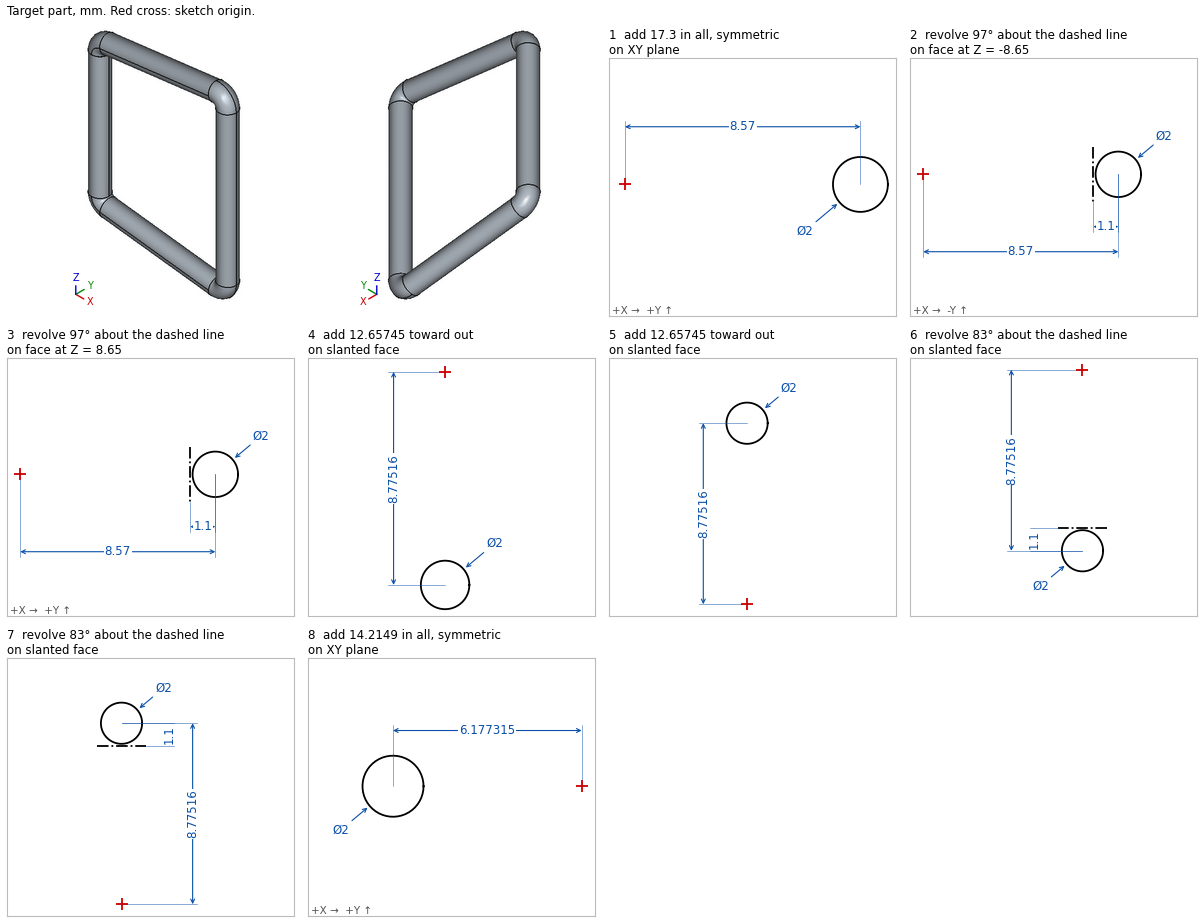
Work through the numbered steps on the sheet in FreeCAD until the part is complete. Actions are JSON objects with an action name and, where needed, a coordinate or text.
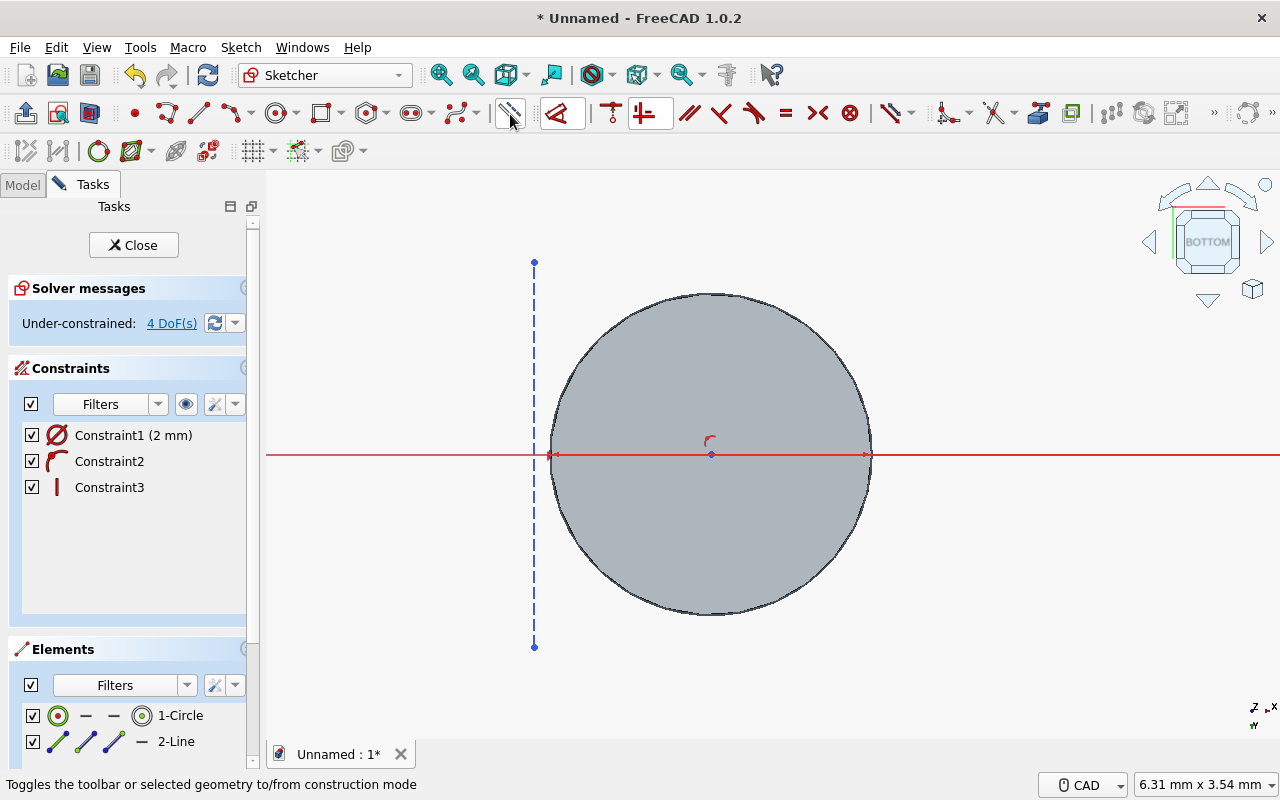
{"action": "left_click", "coordinate": [556, 114]}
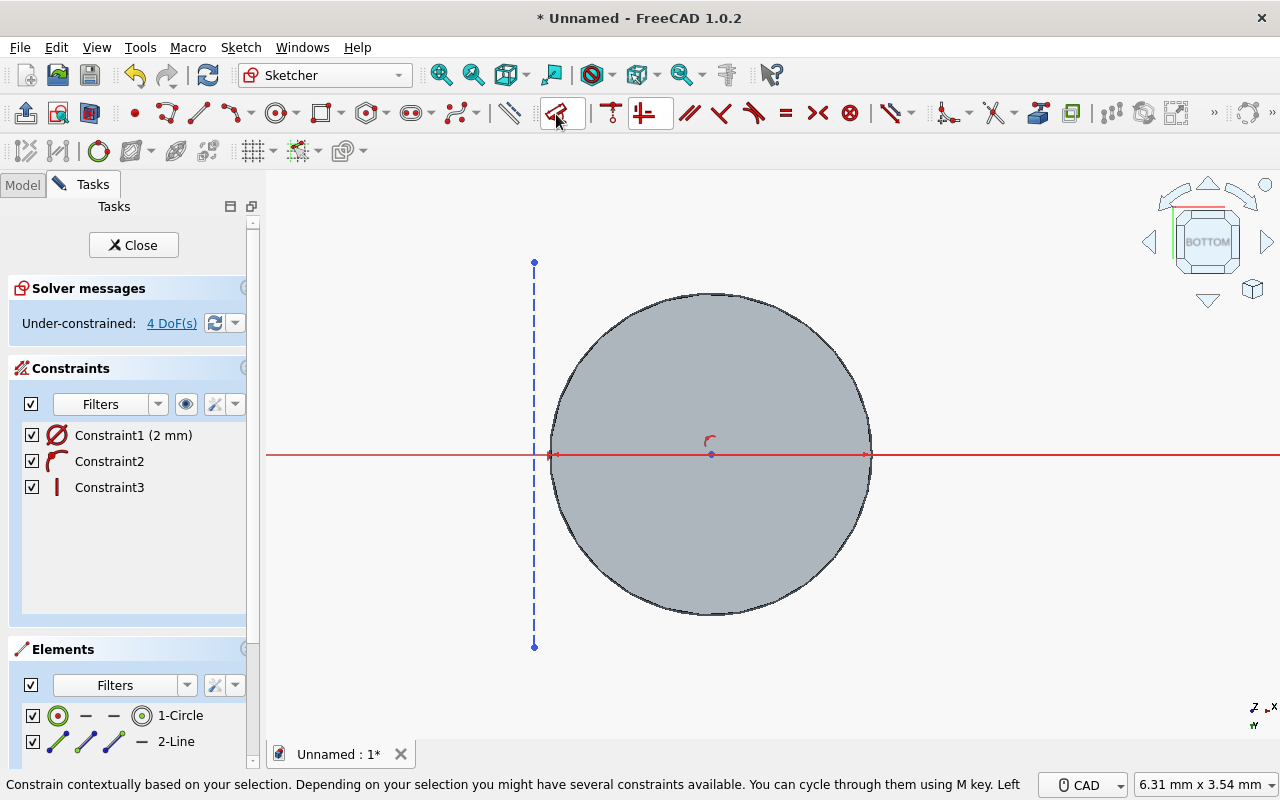
{"action": "scroll", "coordinate": [711, 454], "scroll_direction": "up", "scroll_amount": 4}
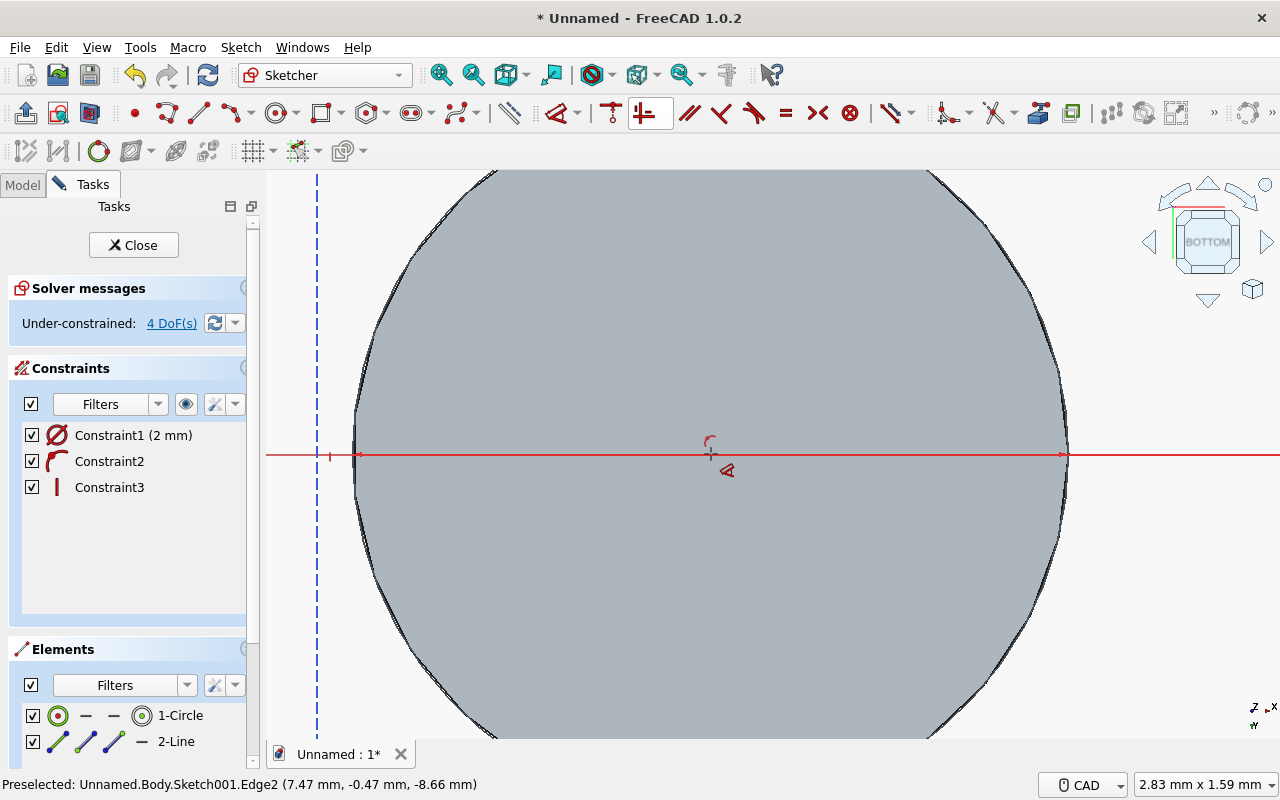
{"action": "left_click", "coordinate": [710, 454]}
{"action": "left_click", "coordinate": [502, 488]}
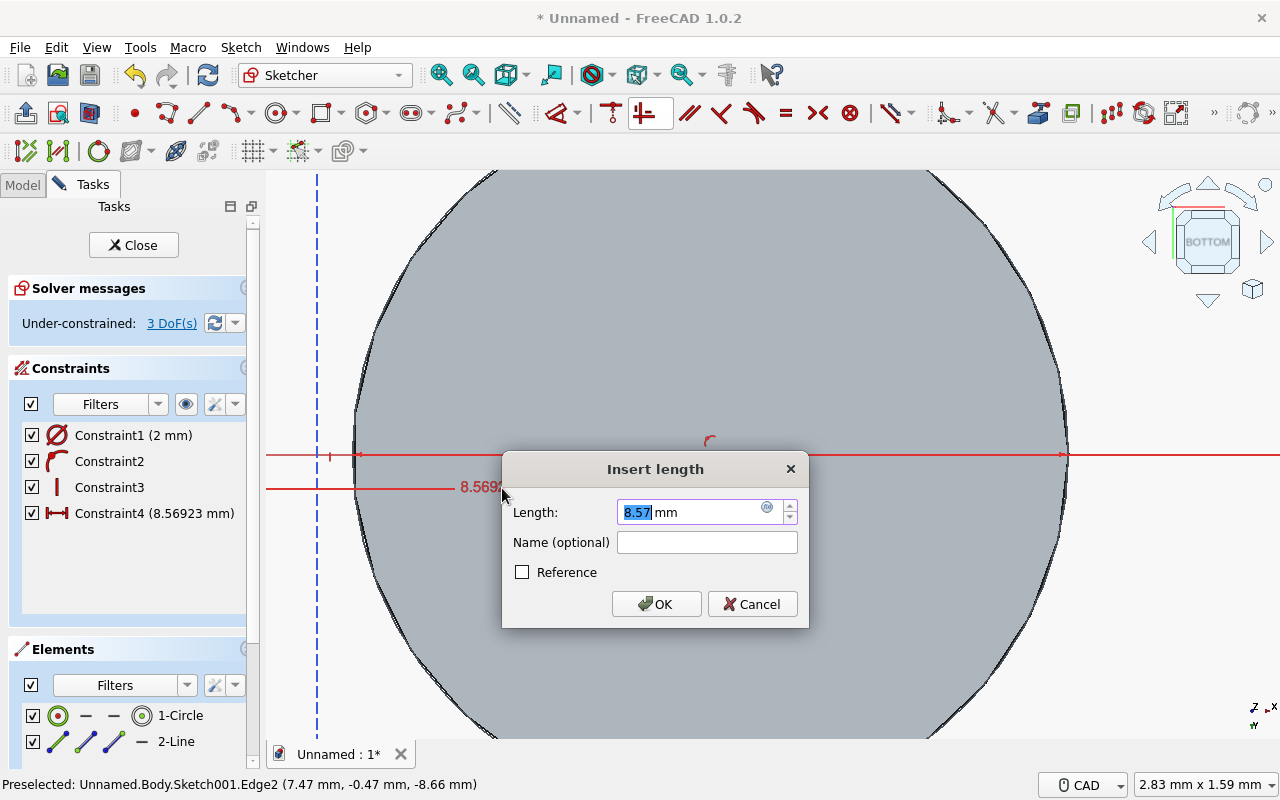
{"action": "type", "text": "8.57"}
{"action": "key", "text": "Return"}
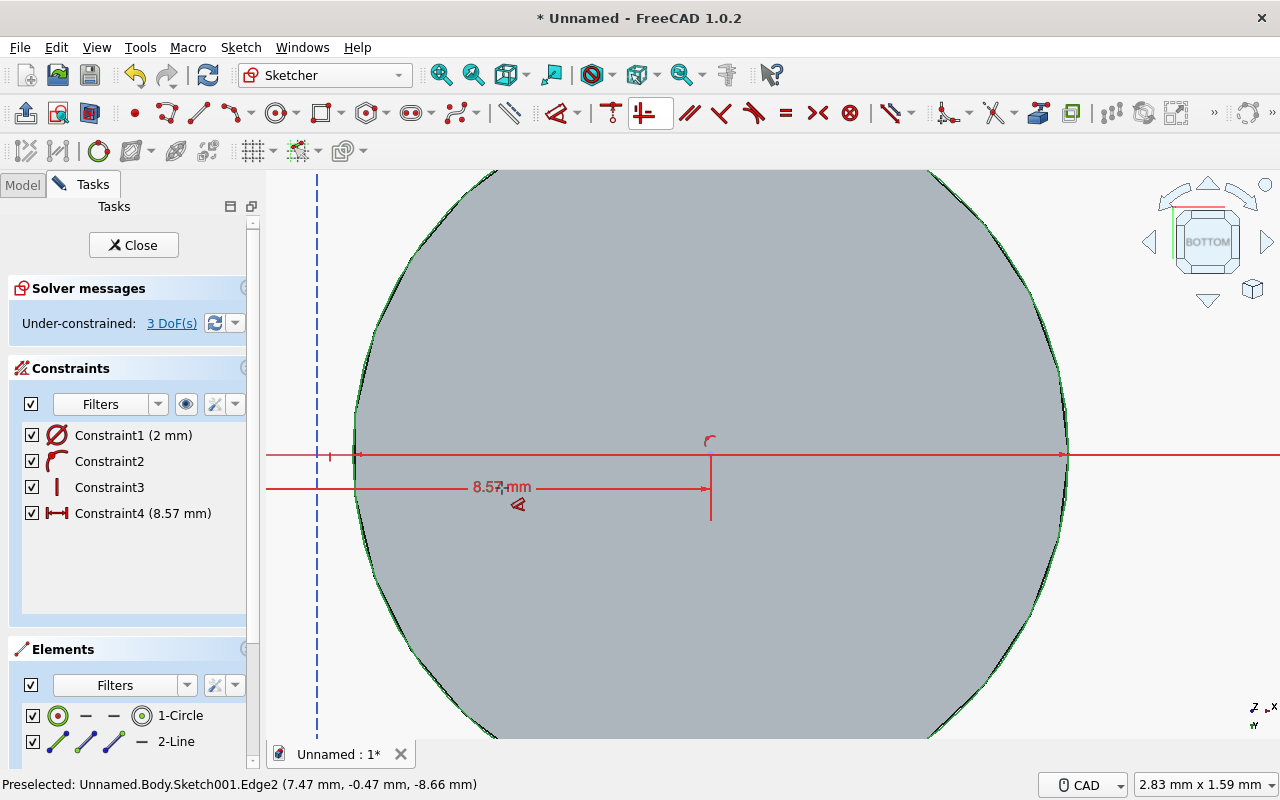
{"action": "scroll", "coordinate": [714, 454], "scroll_direction": "down", "scroll_amount": 4}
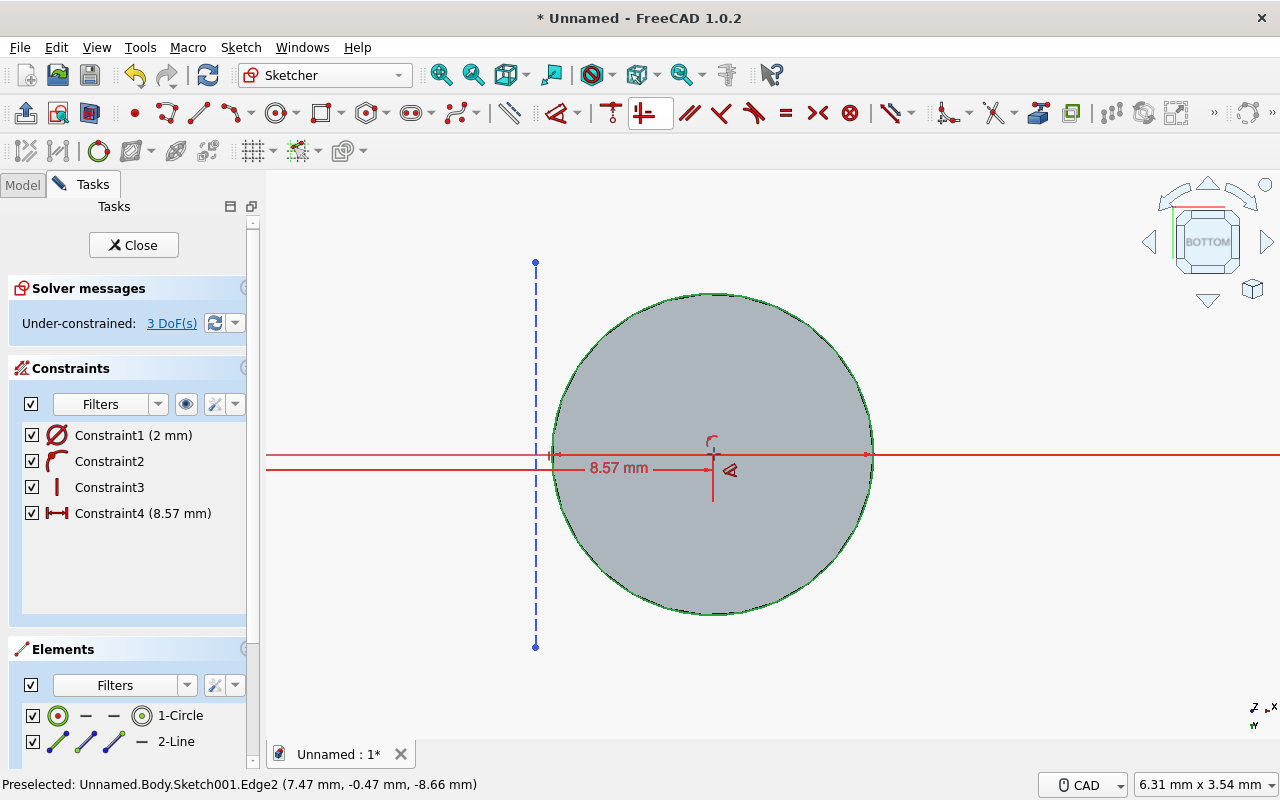
{"action": "left_click", "coordinate": [538, 650]}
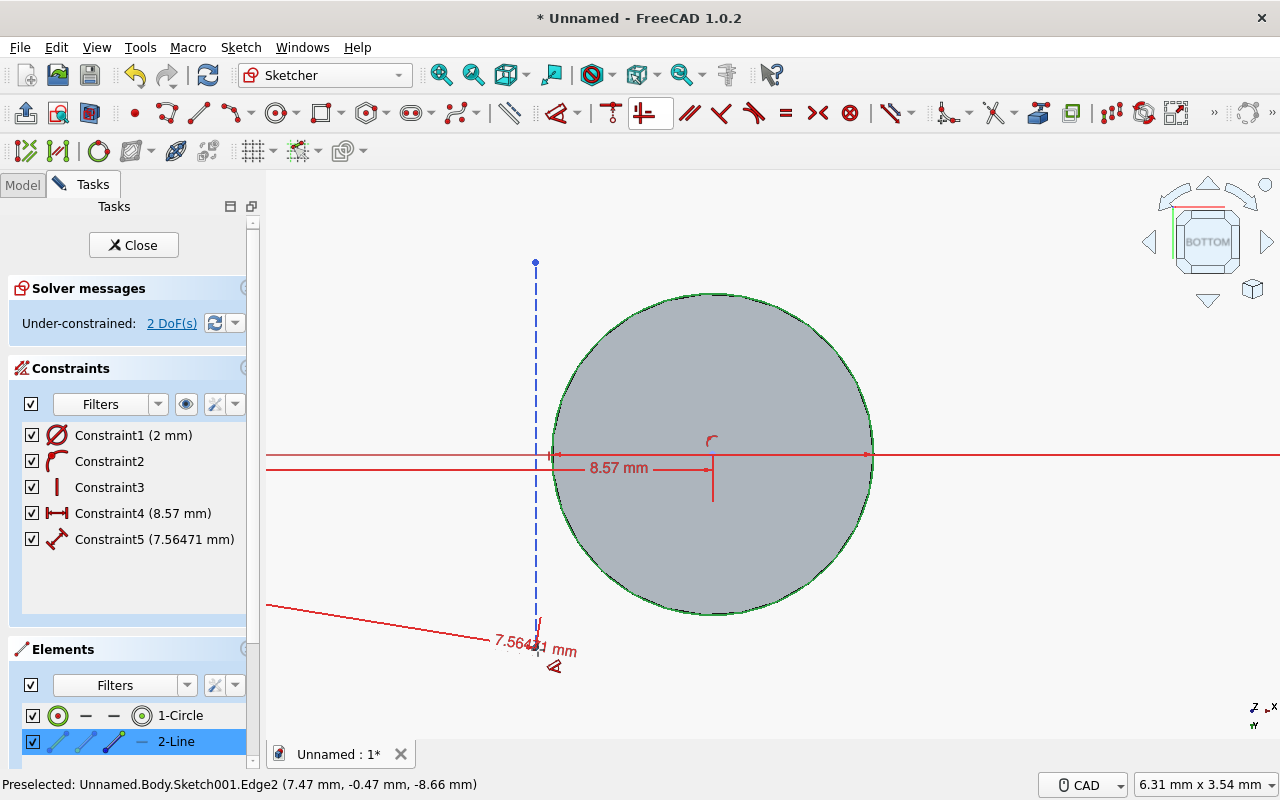
{"action": "left_click", "coordinate": [713, 454]}
{"action": "left_click", "coordinate": [624, 682]}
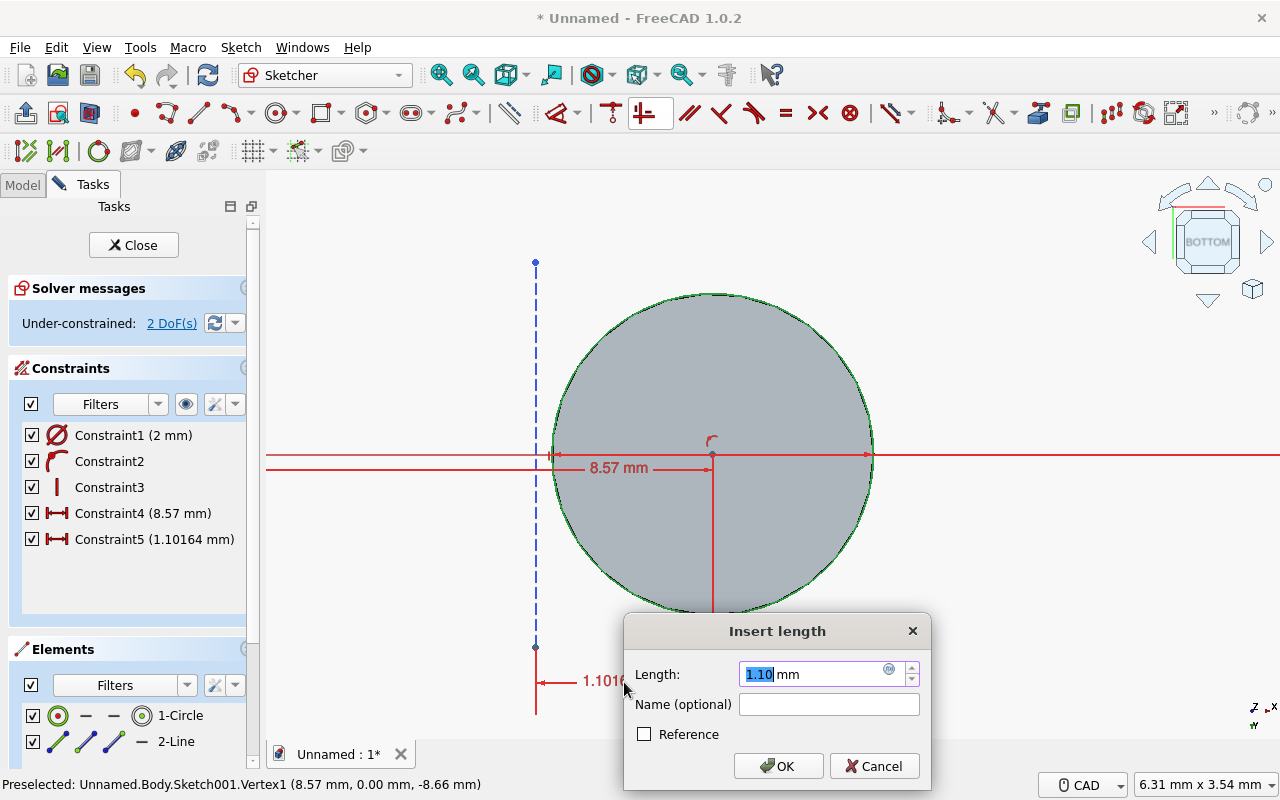
{"action": "type", "text": "1.1"}
{"action": "key", "text": "Return"}
{"action": "key", "text": "Escape"}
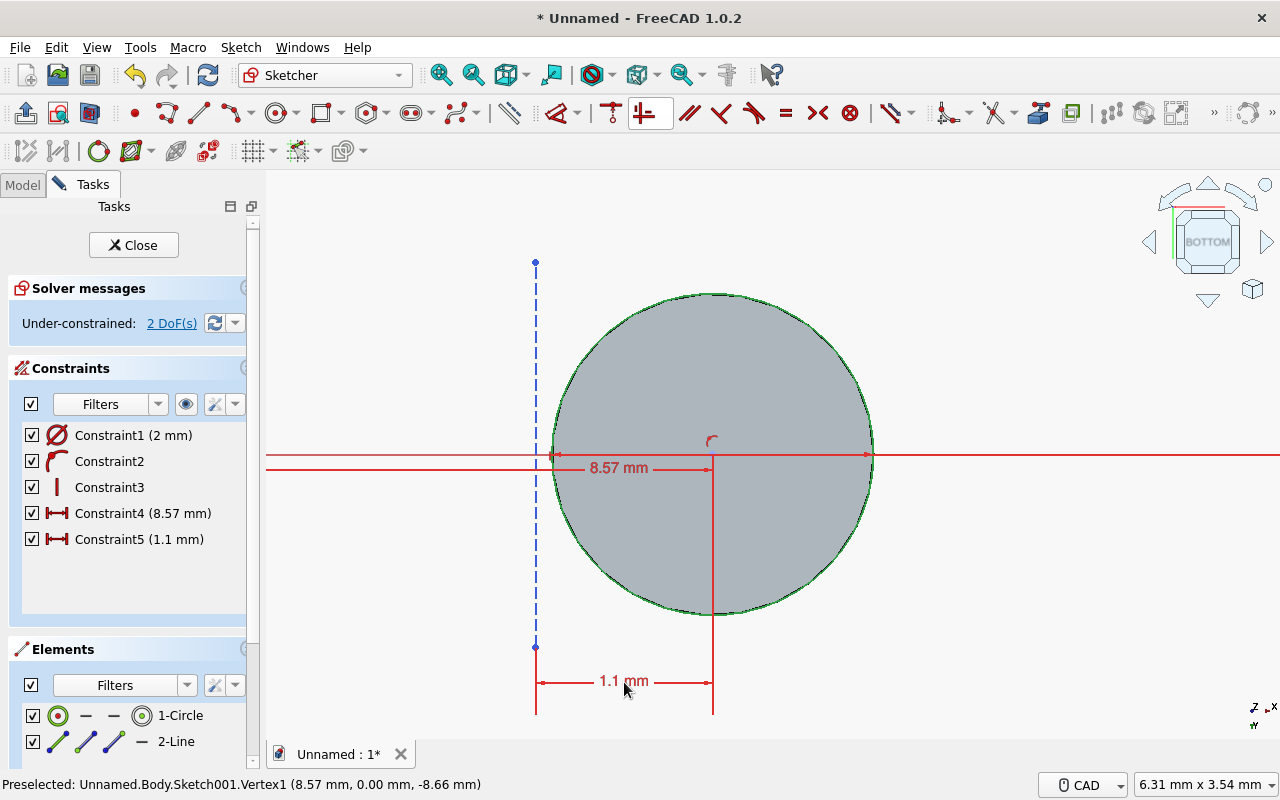
{"action": "left_click", "coordinate": [134, 245]}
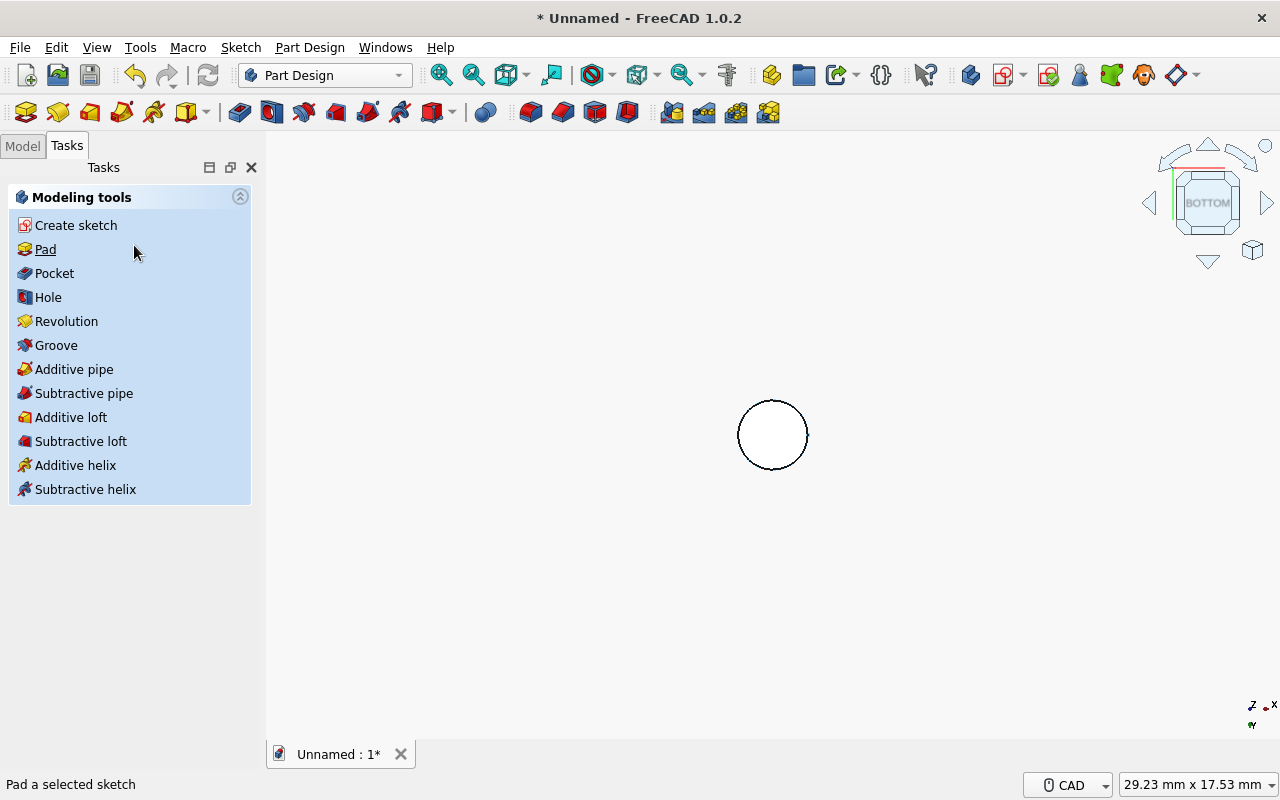
{"action": "left_click", "coordinate": [58, 112]}